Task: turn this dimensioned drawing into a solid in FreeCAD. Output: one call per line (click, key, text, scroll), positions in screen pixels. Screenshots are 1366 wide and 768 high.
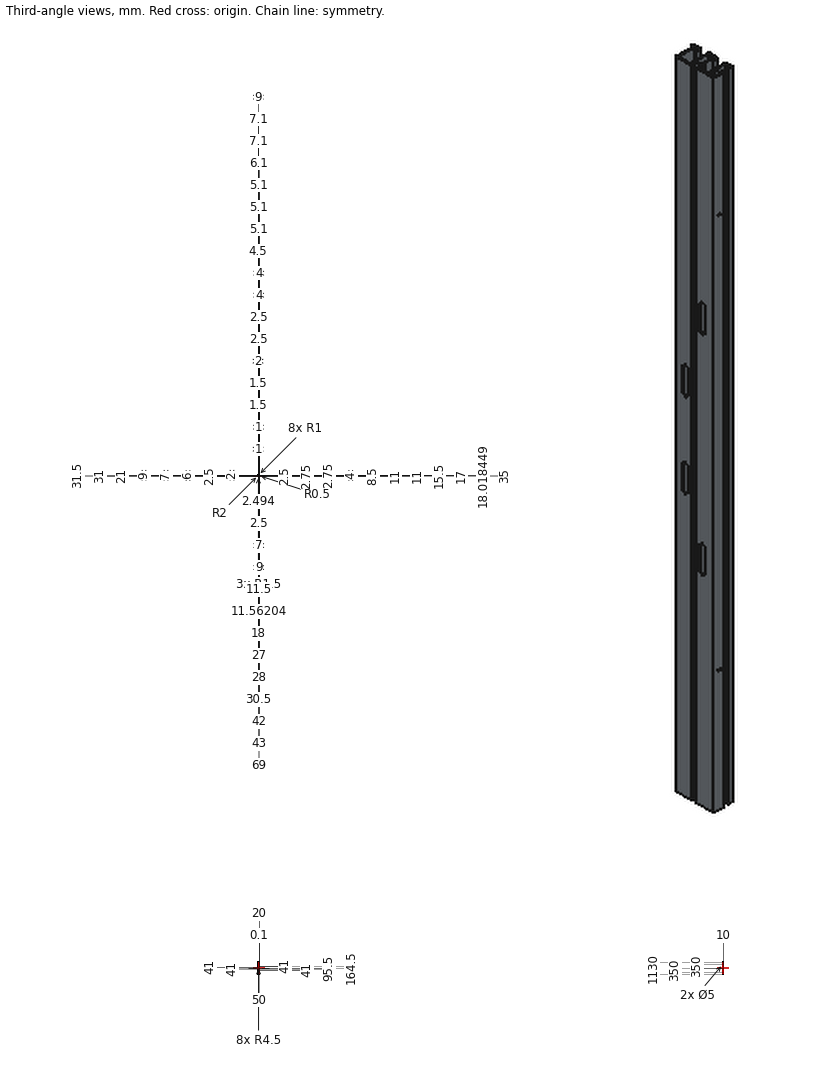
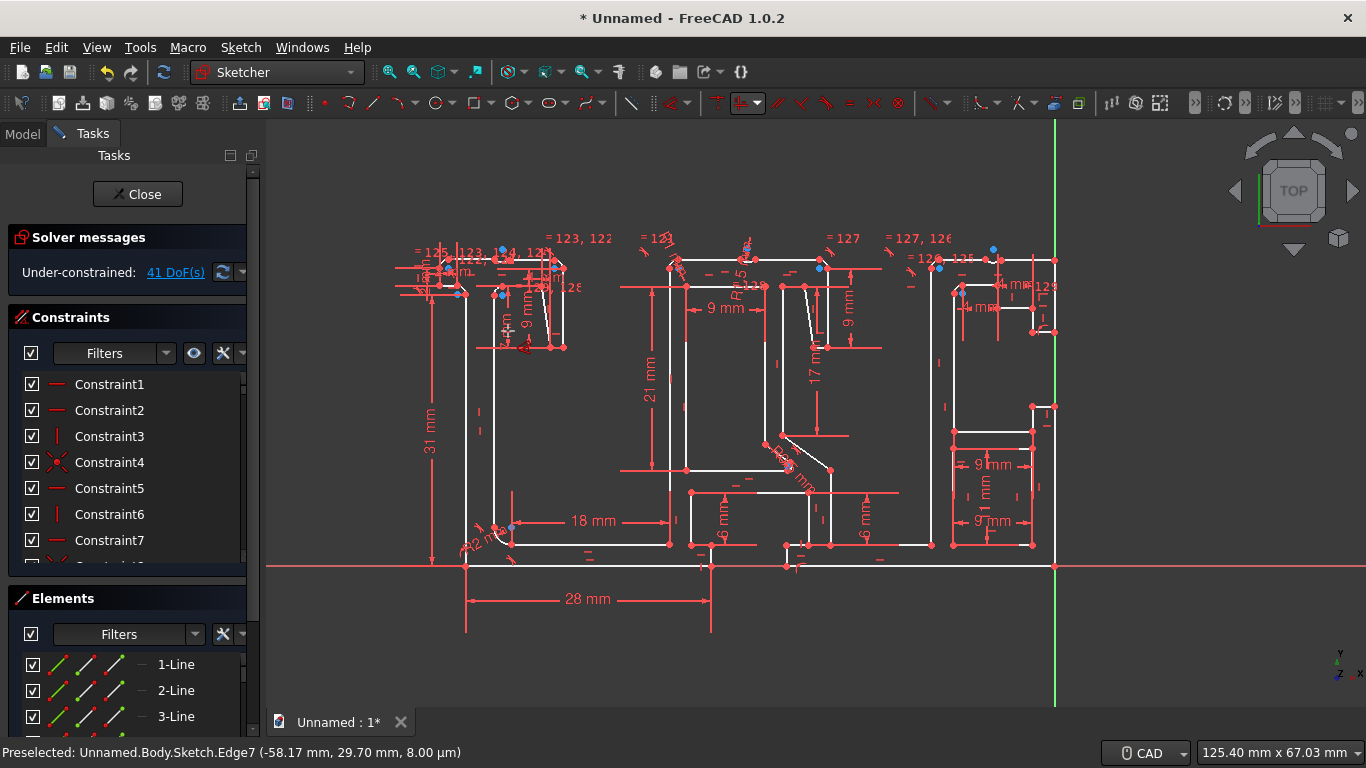
click(816, 460)
click(865, 453)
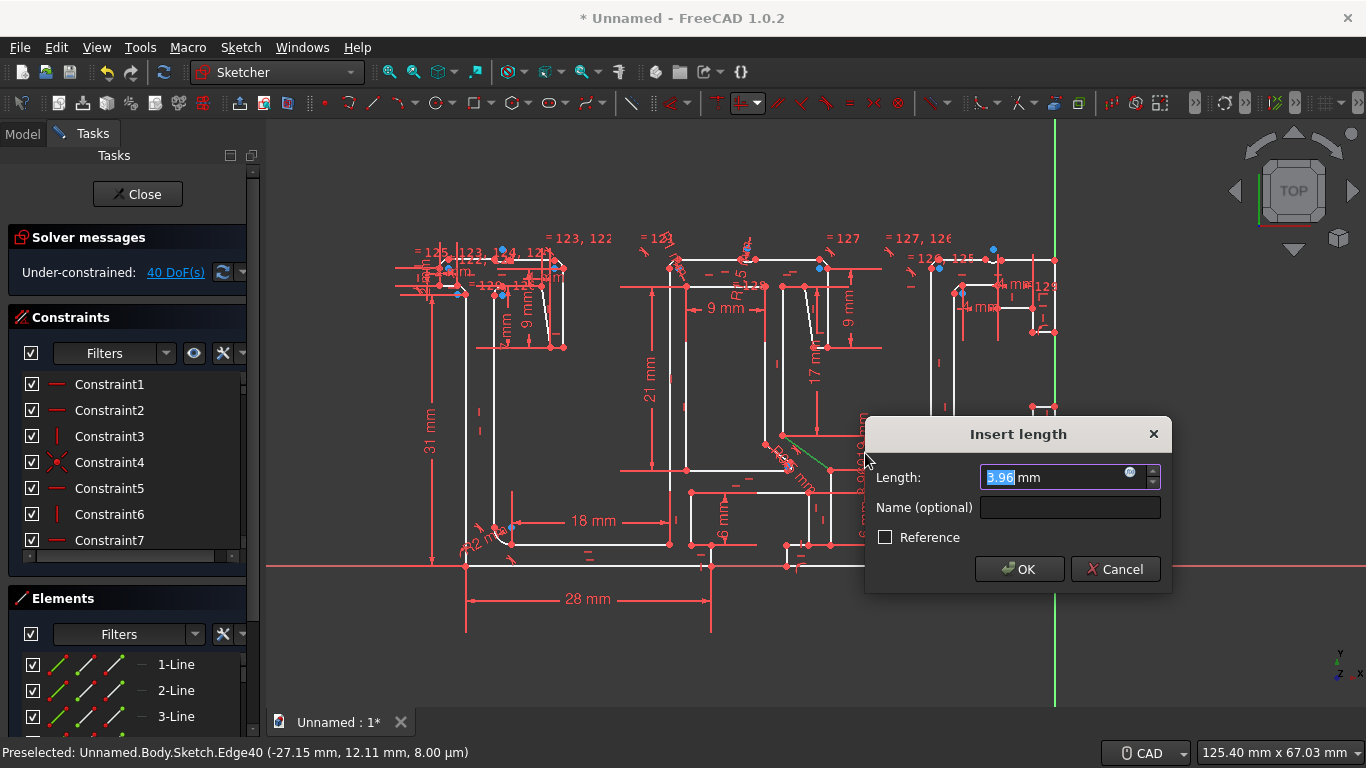
text(4)
key(Return)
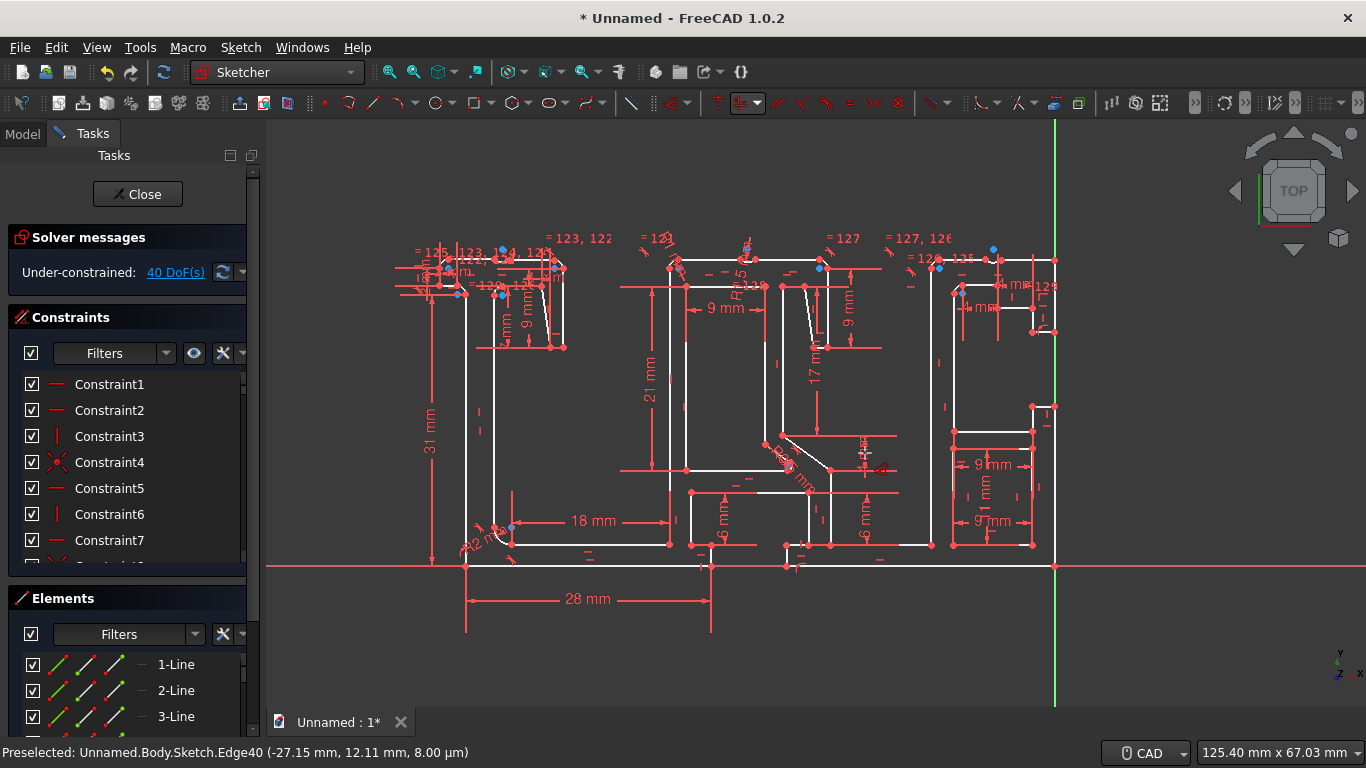
scroll(807, 305, up, 8)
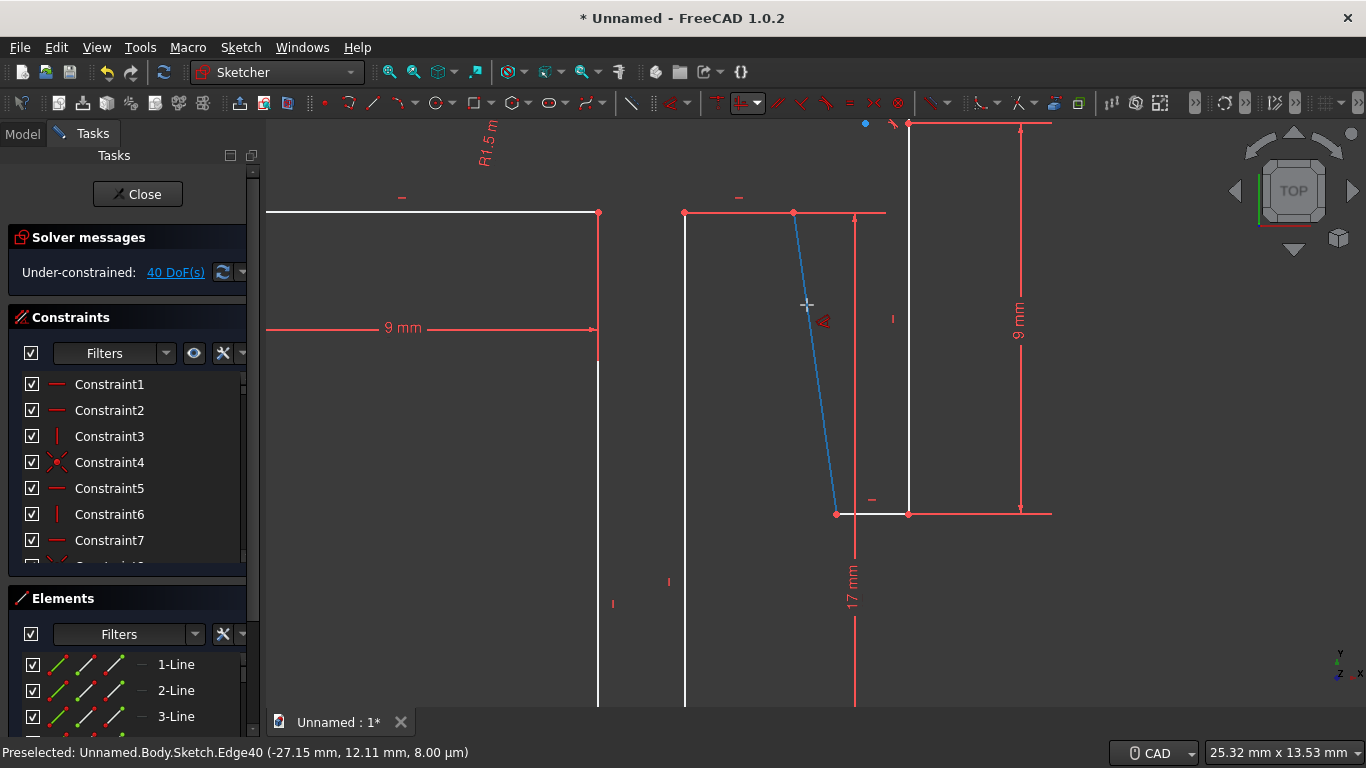
click(807, 303)
click(815, 179)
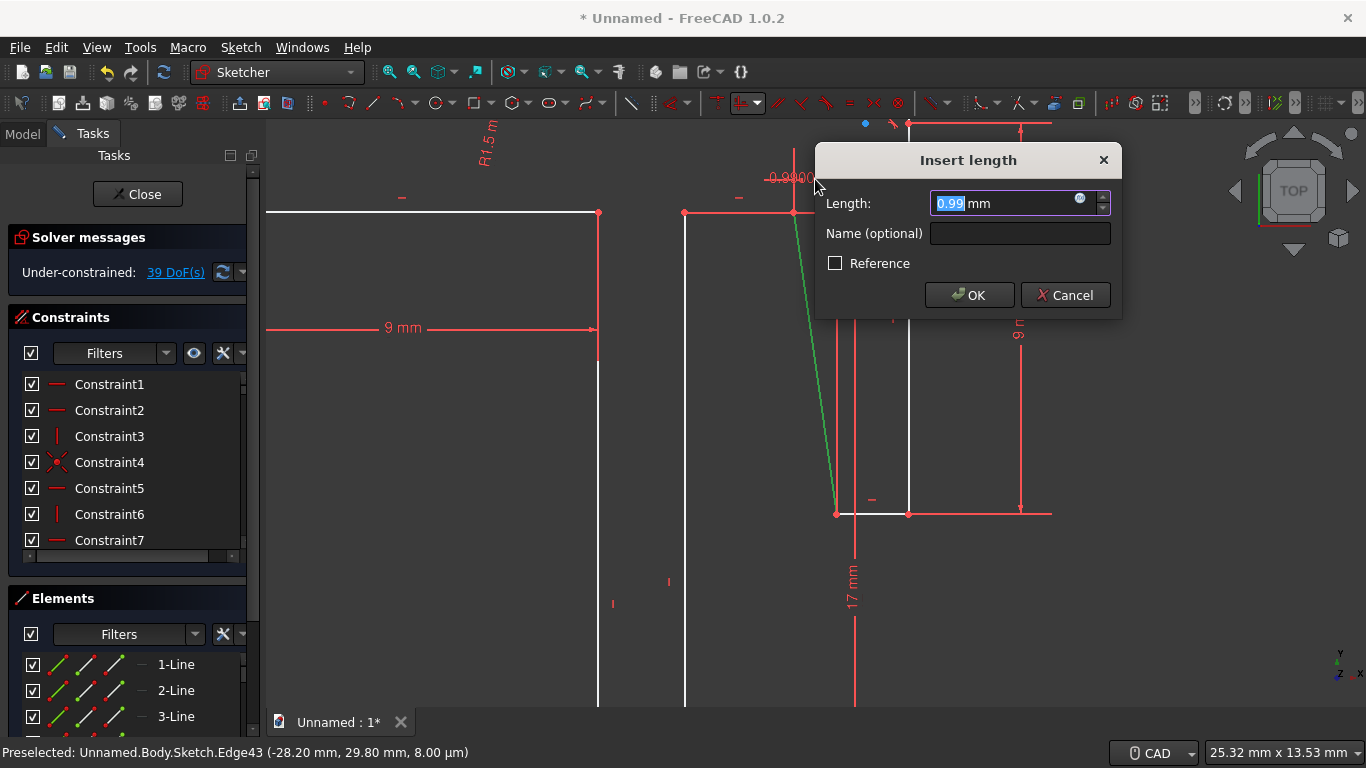
text(1)
key(Return)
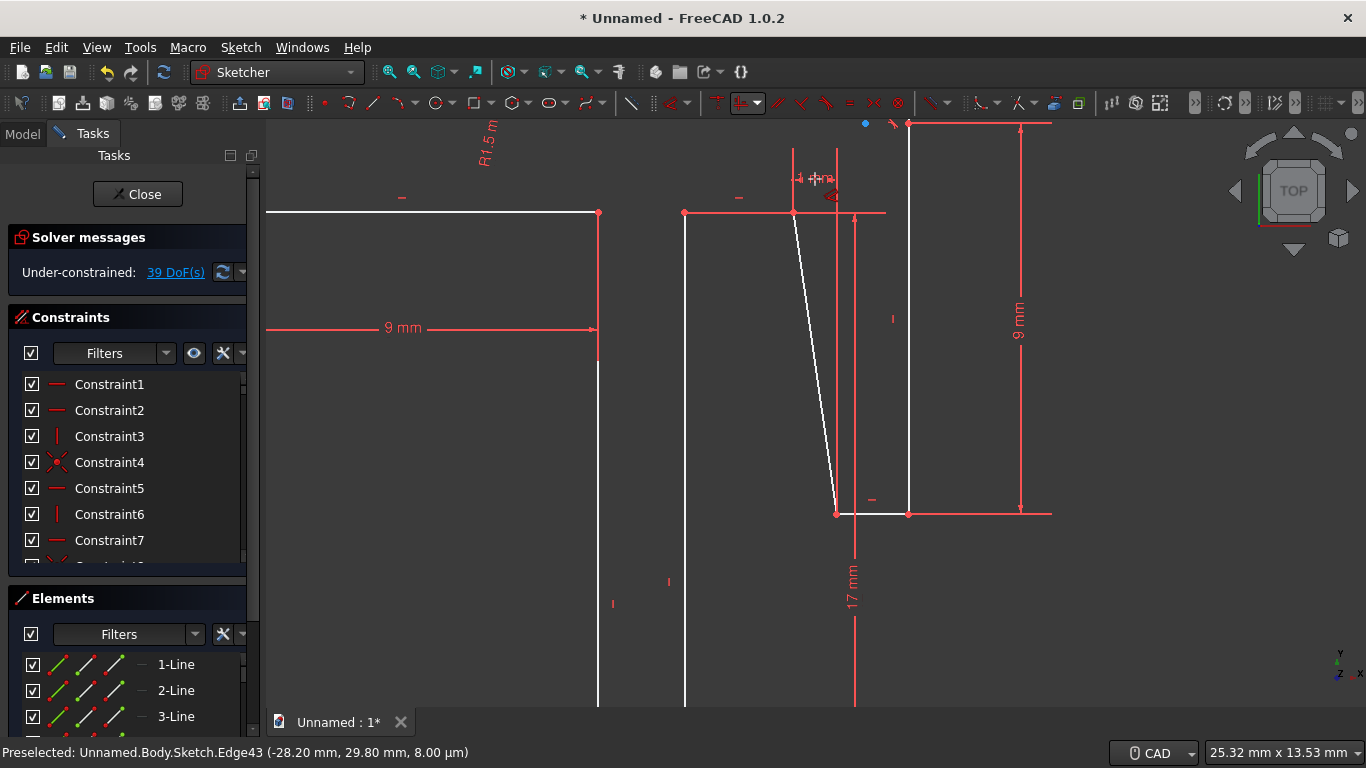
scroll(807, 305, down, 8)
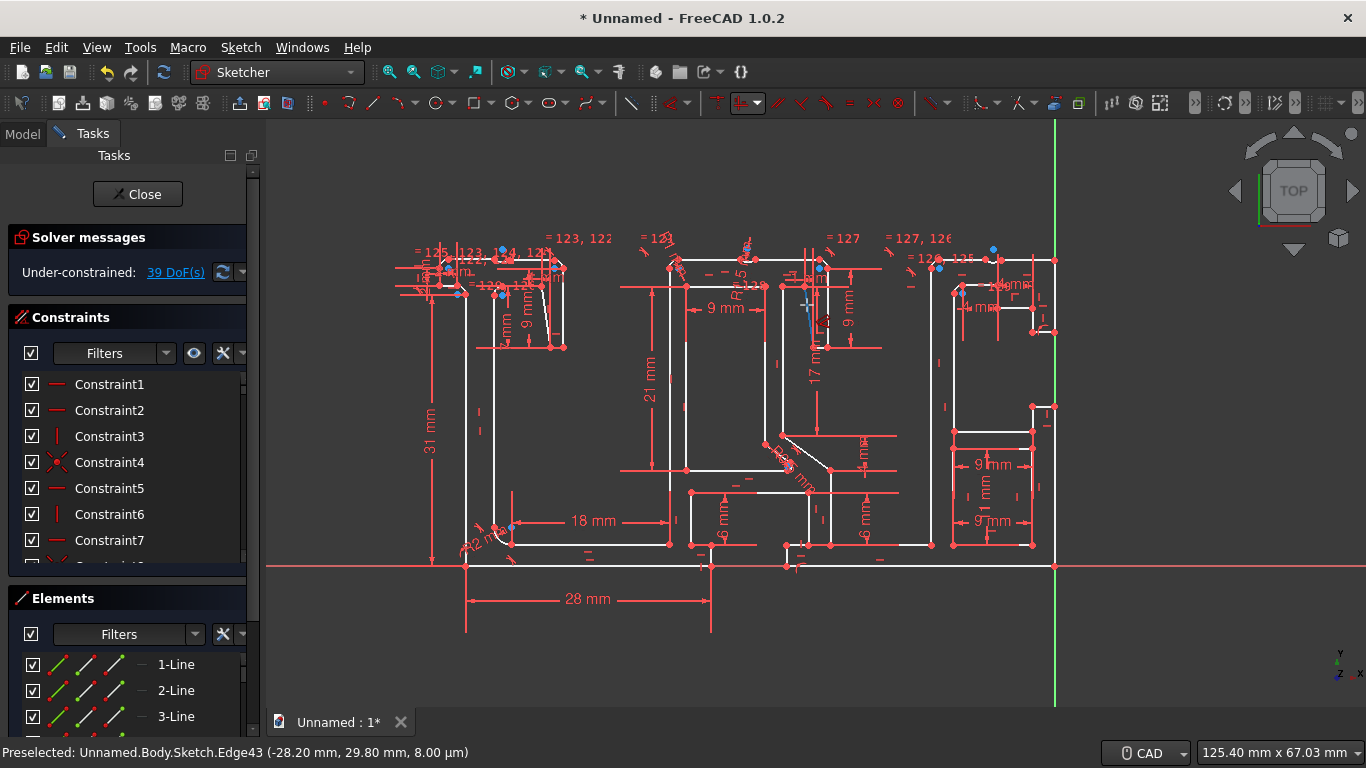
click(807, 305)
click(847, 331)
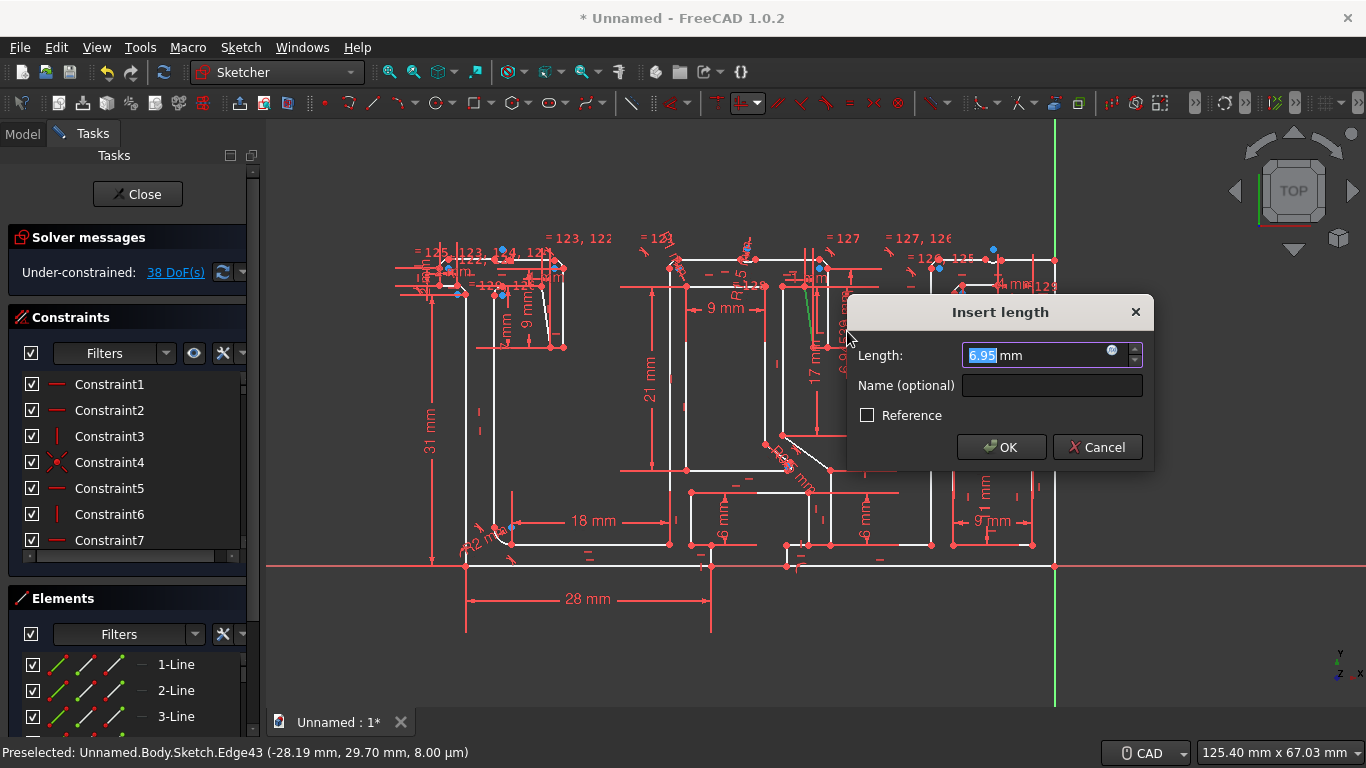
text(7)
key(Return)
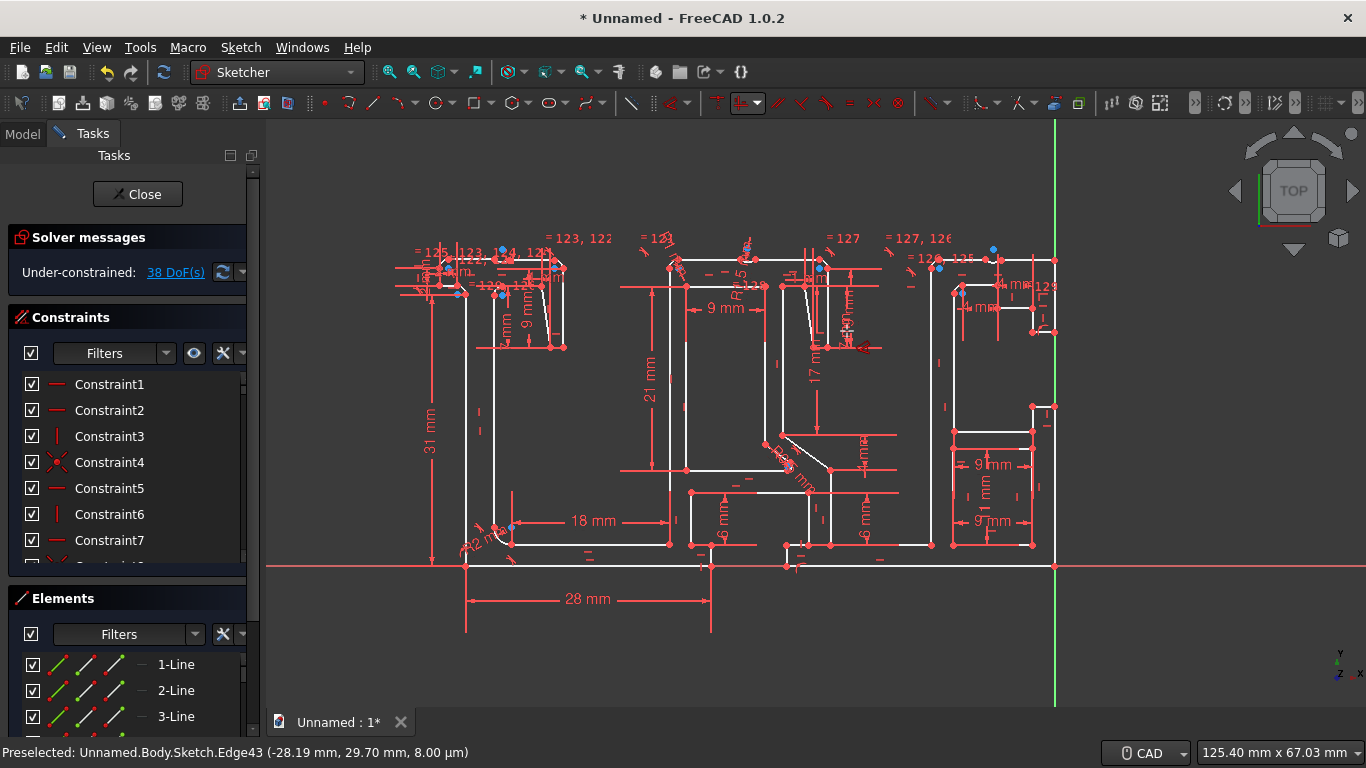
click(993, 249)
click(1024, 215)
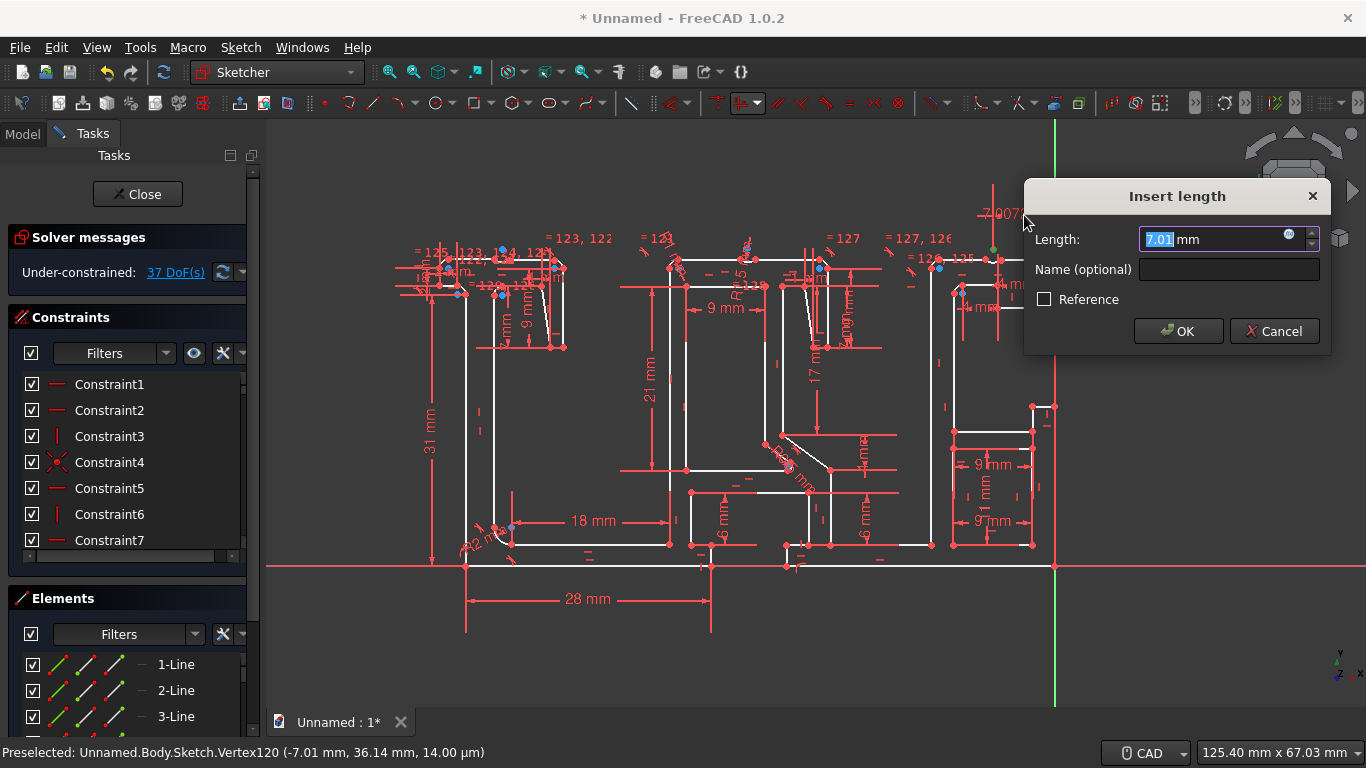
text(7)
key(Return)